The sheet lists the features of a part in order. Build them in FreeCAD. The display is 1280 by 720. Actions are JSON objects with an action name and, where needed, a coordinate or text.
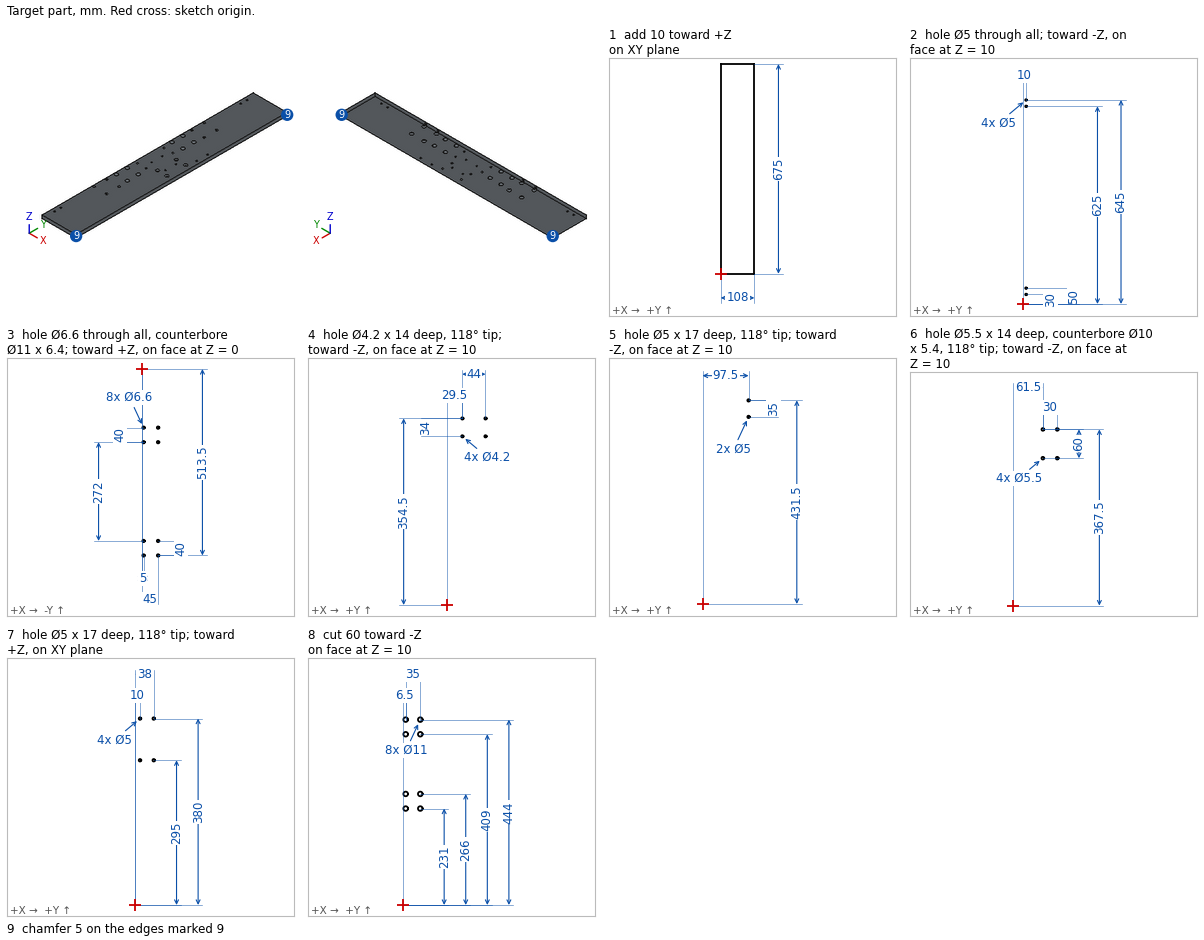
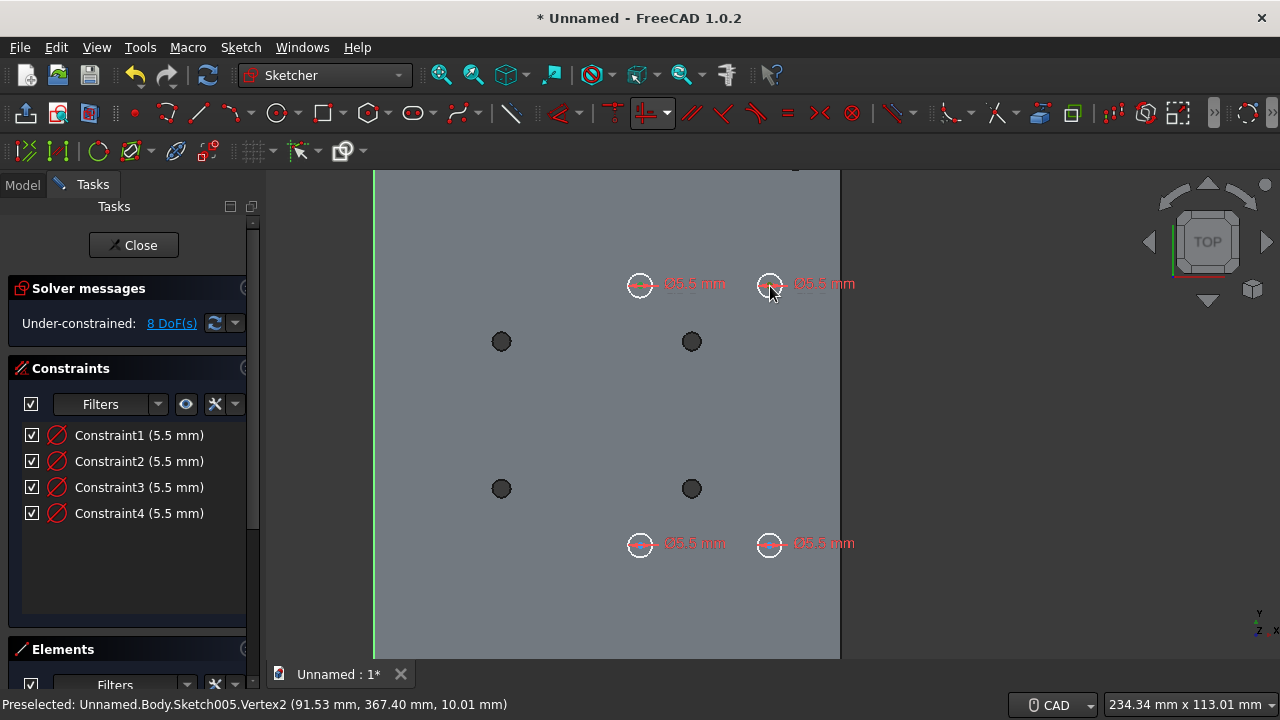
{"action": "key", "text": "h"}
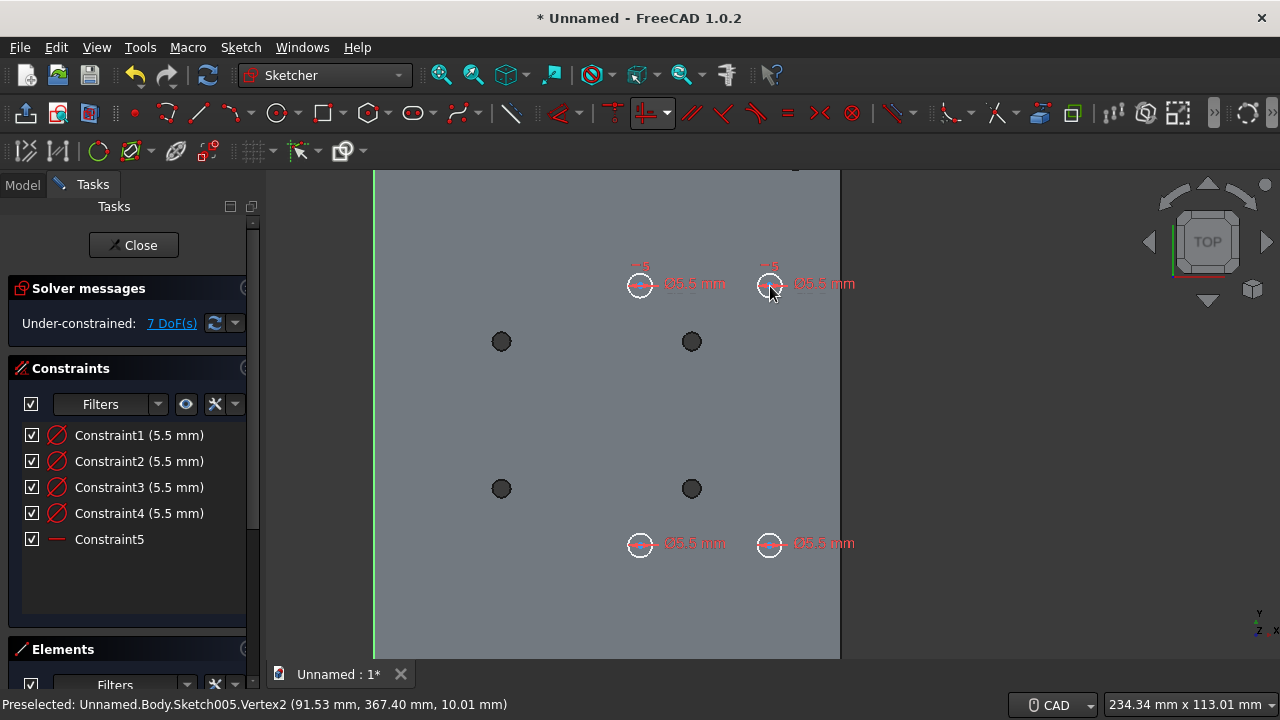
{"action": "left_click", "coordinate": [640, 286]}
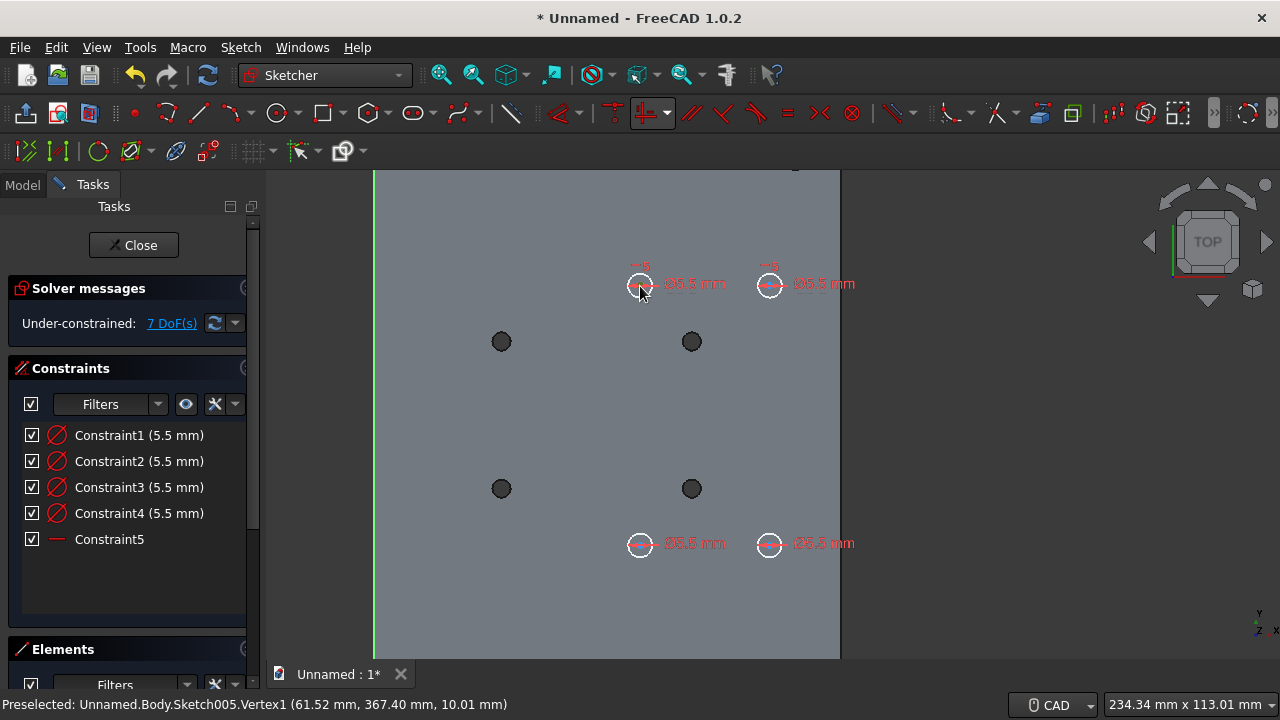
{"action": "left_click", "coordinate": [640, 545]}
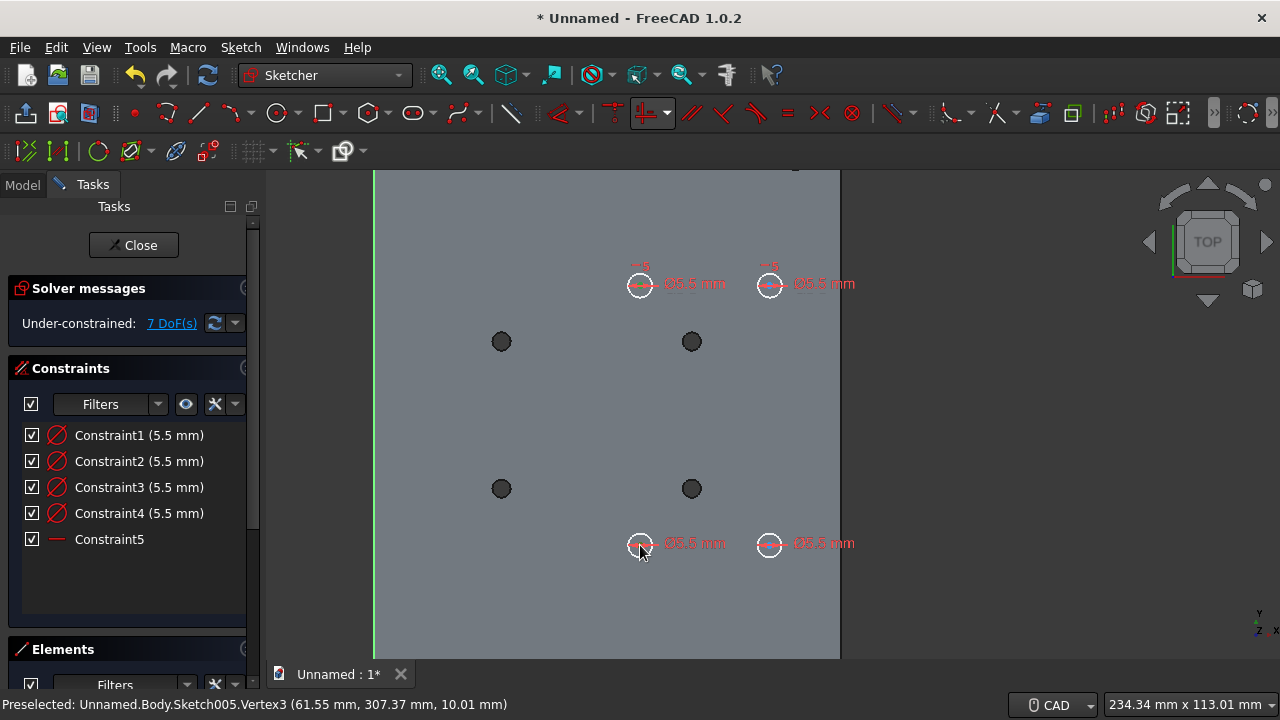
{"action": "left_click", "coordinate": [670, 114]}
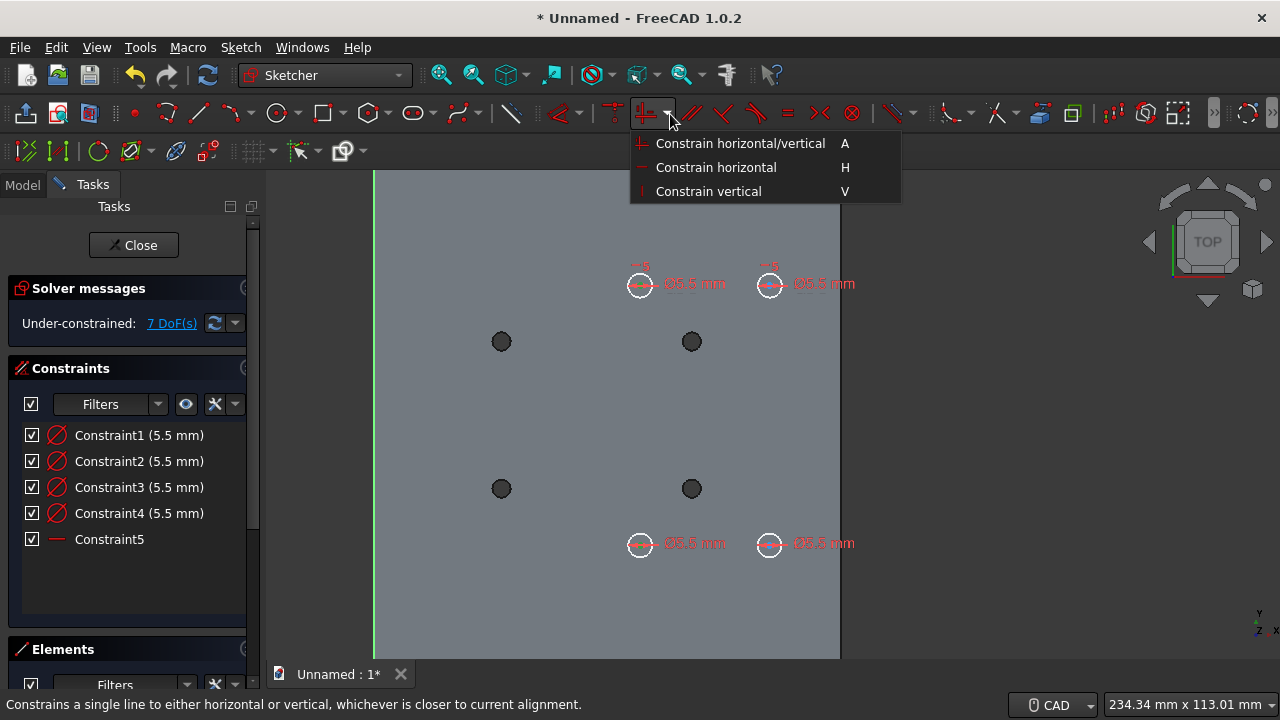
{"action": "left_click", "coordinate": [766, 191]}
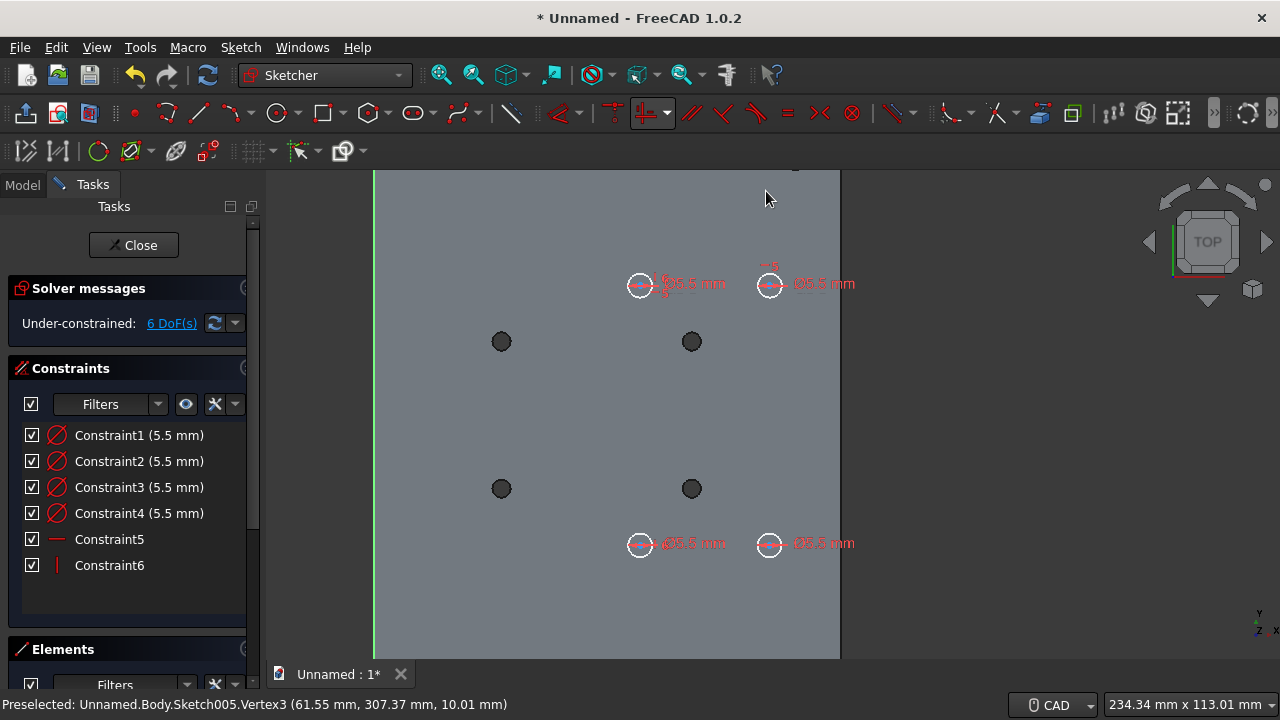
{"action": "left_click", "coordinate": [770, 286]}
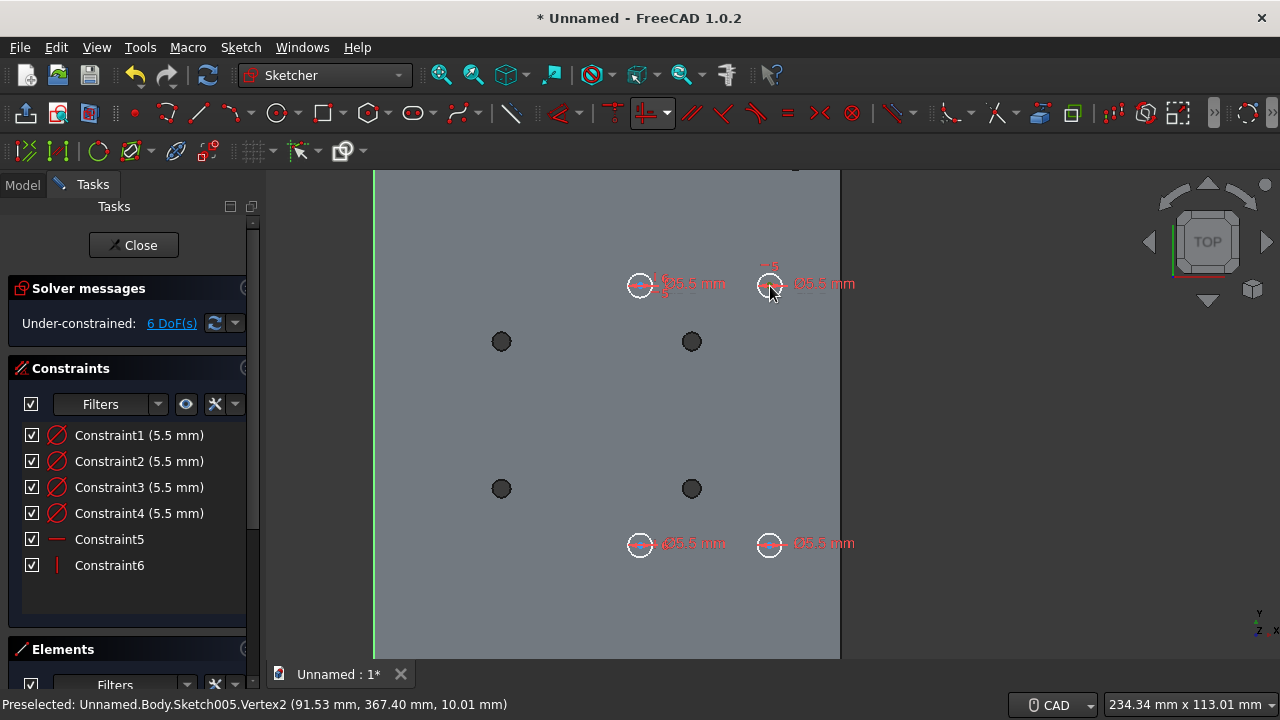
{"action": "left_click", "coordinate": [770, 545]}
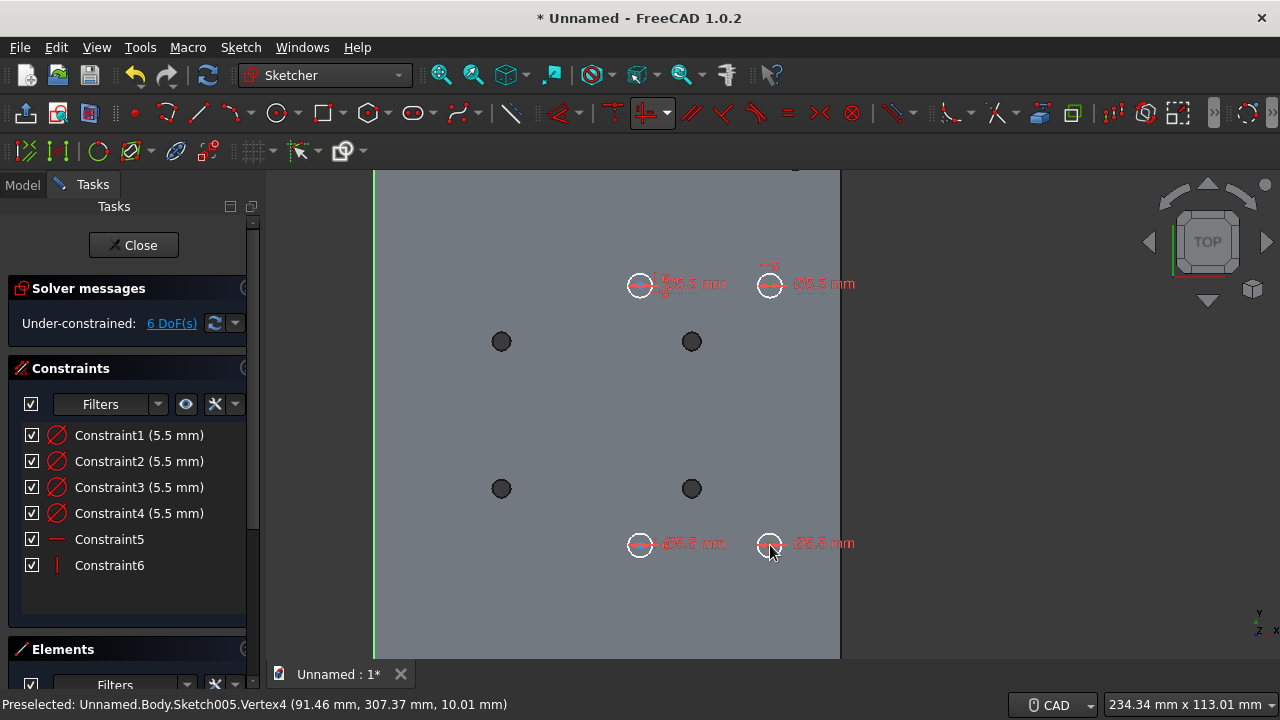
{"action": "left_click", "coordinate": [670, 114]}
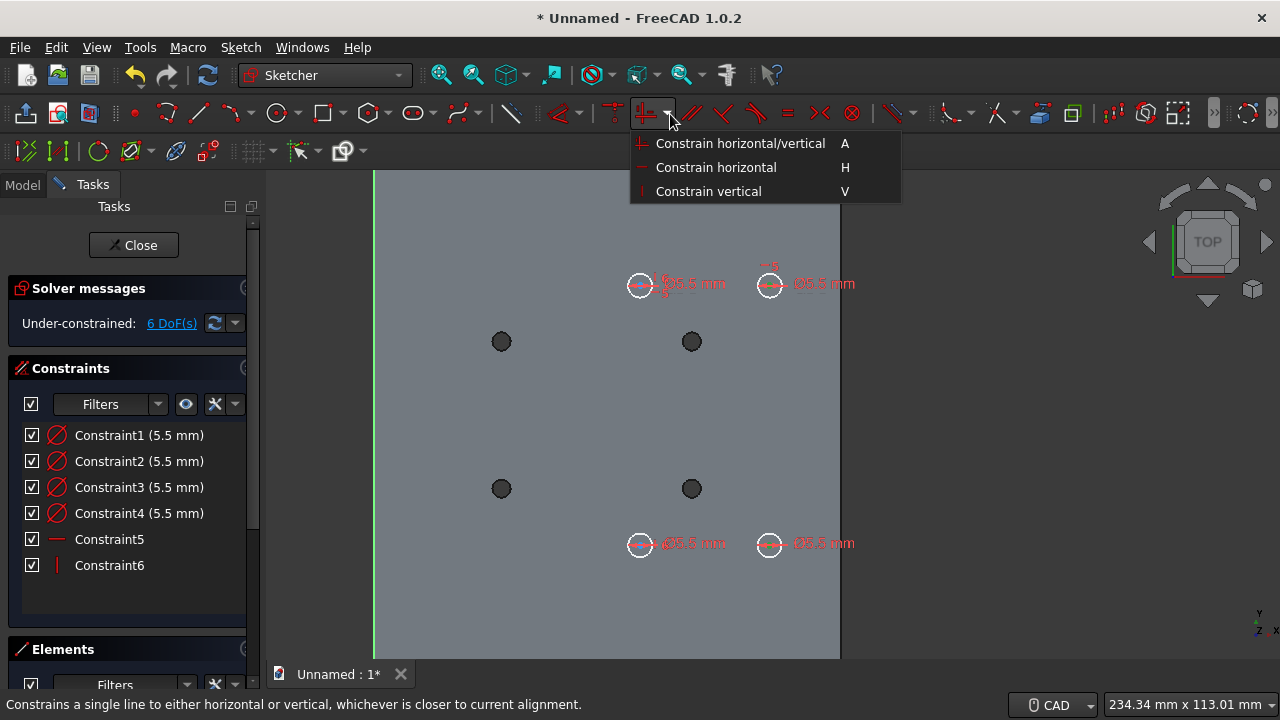
{"action": "left_click", "coordinate": [766, 191]}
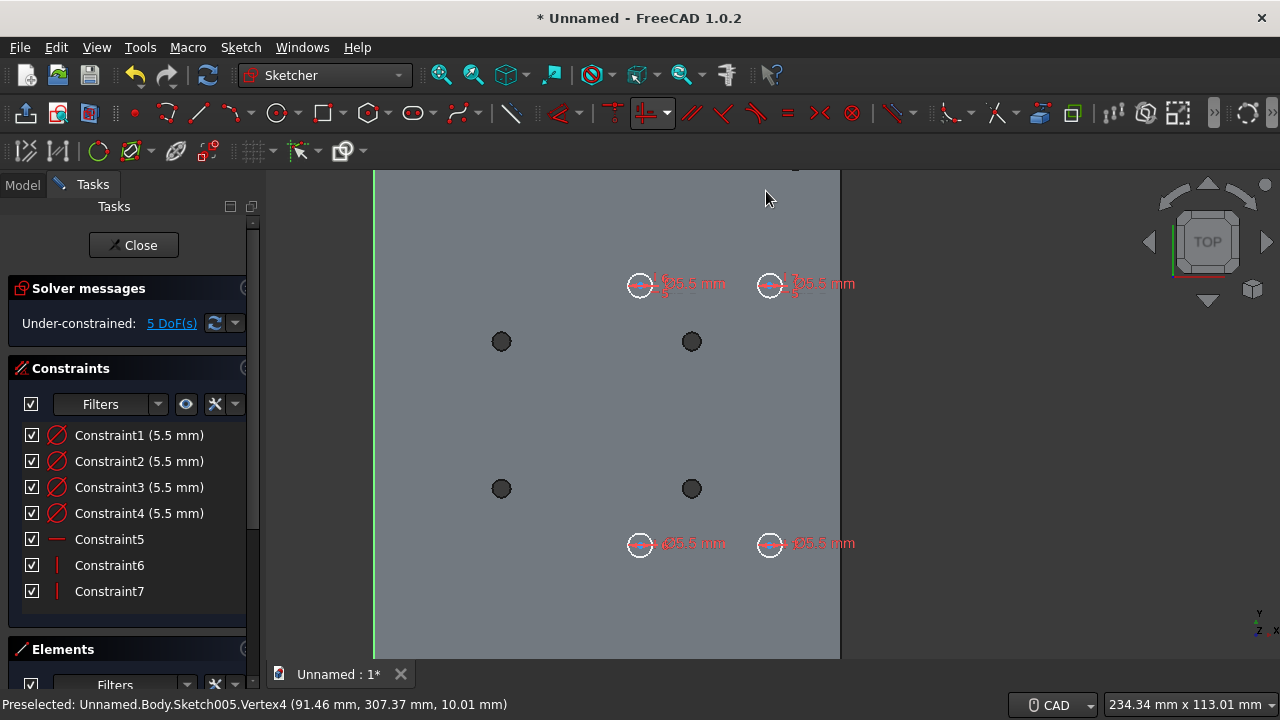
{"action": "left_click", "coordinate": [640, 545]}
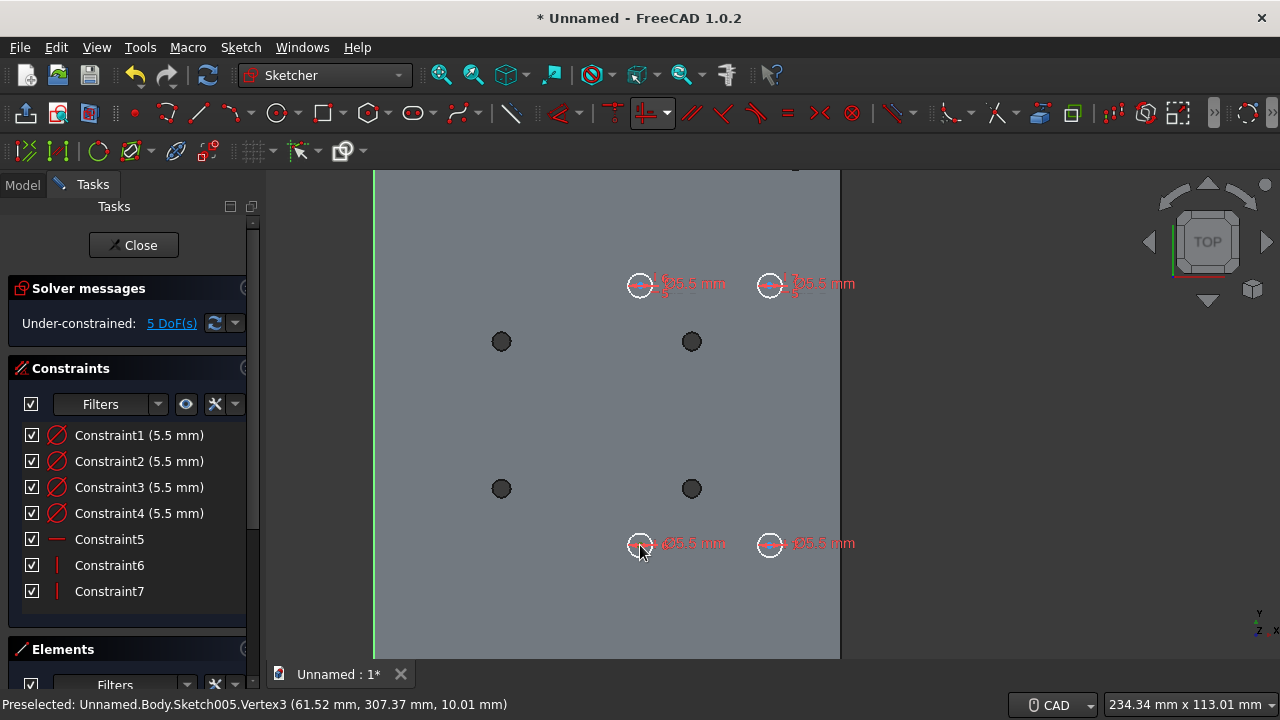
{"action": "left_click", "coordinate": [770, 545]}